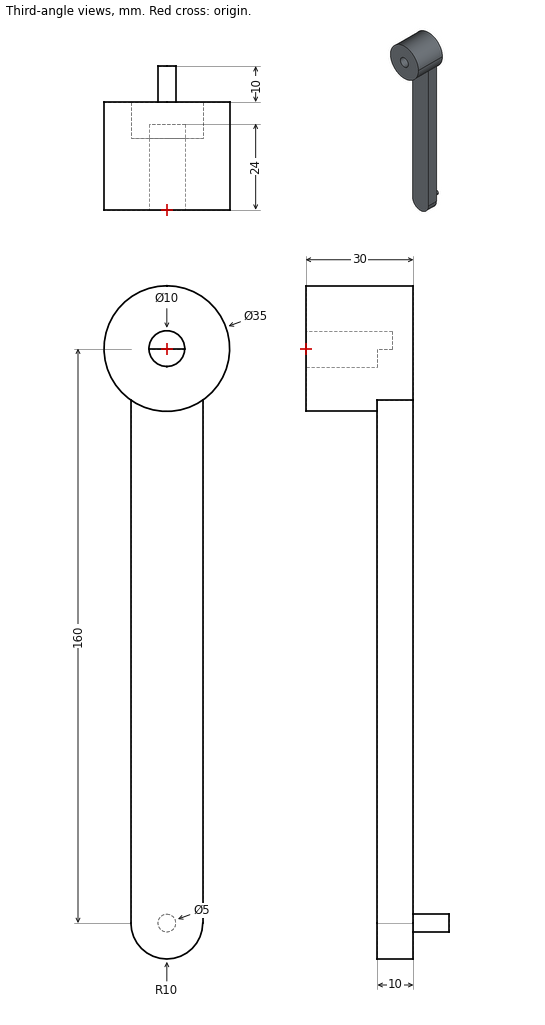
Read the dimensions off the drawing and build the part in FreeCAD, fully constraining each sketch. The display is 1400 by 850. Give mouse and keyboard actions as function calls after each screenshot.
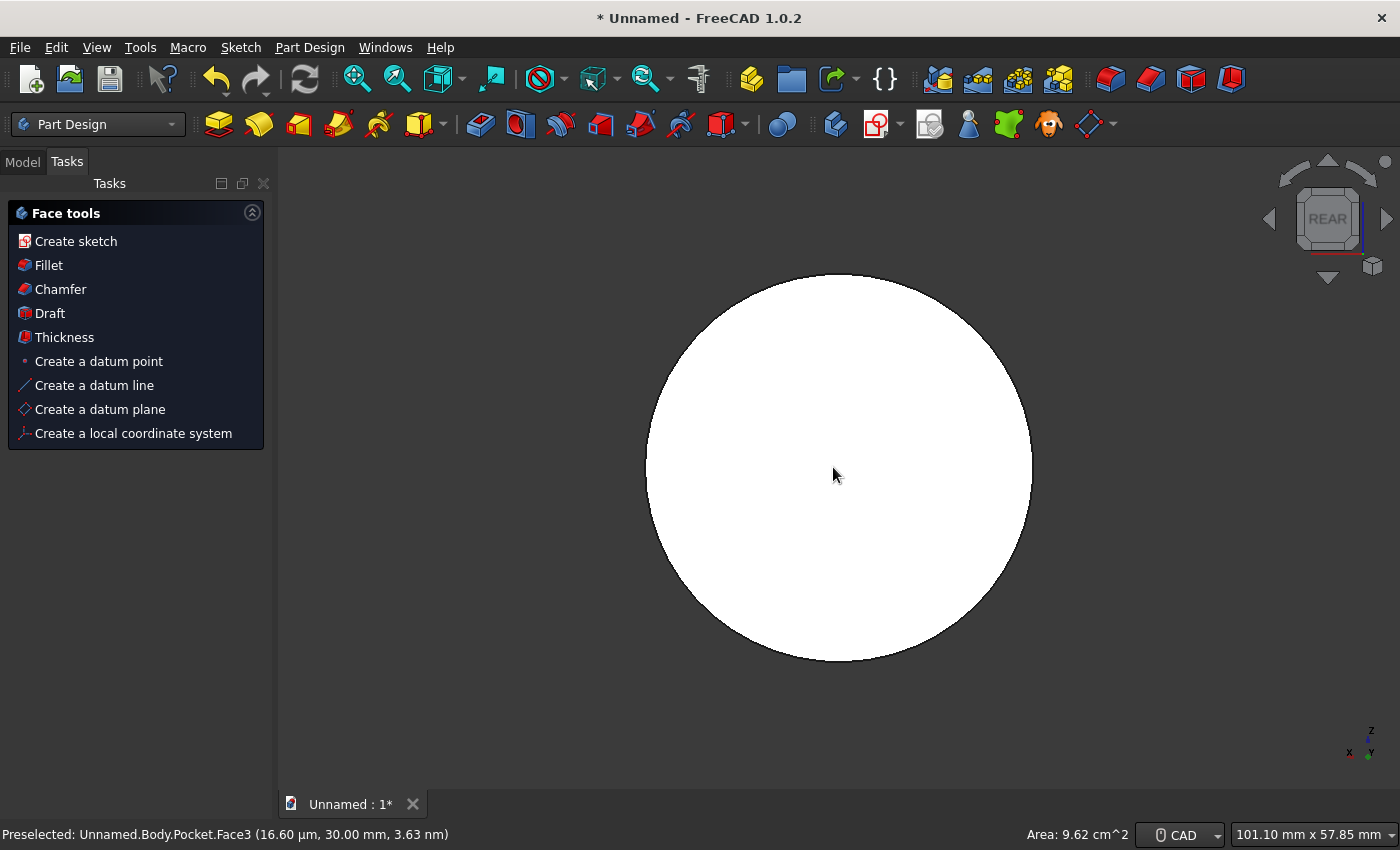
click(876, 124)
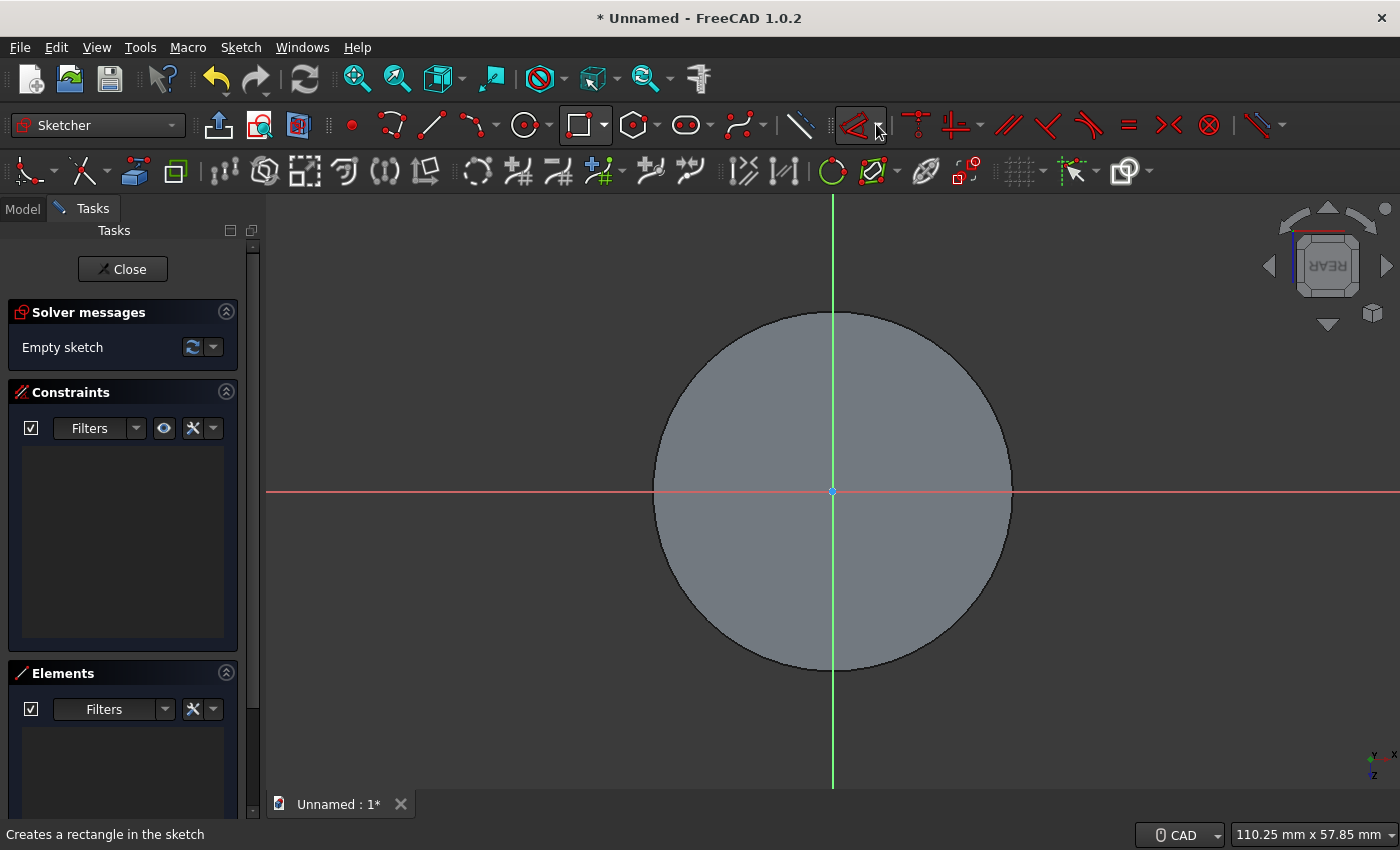
scroll(747, 713, down, 8)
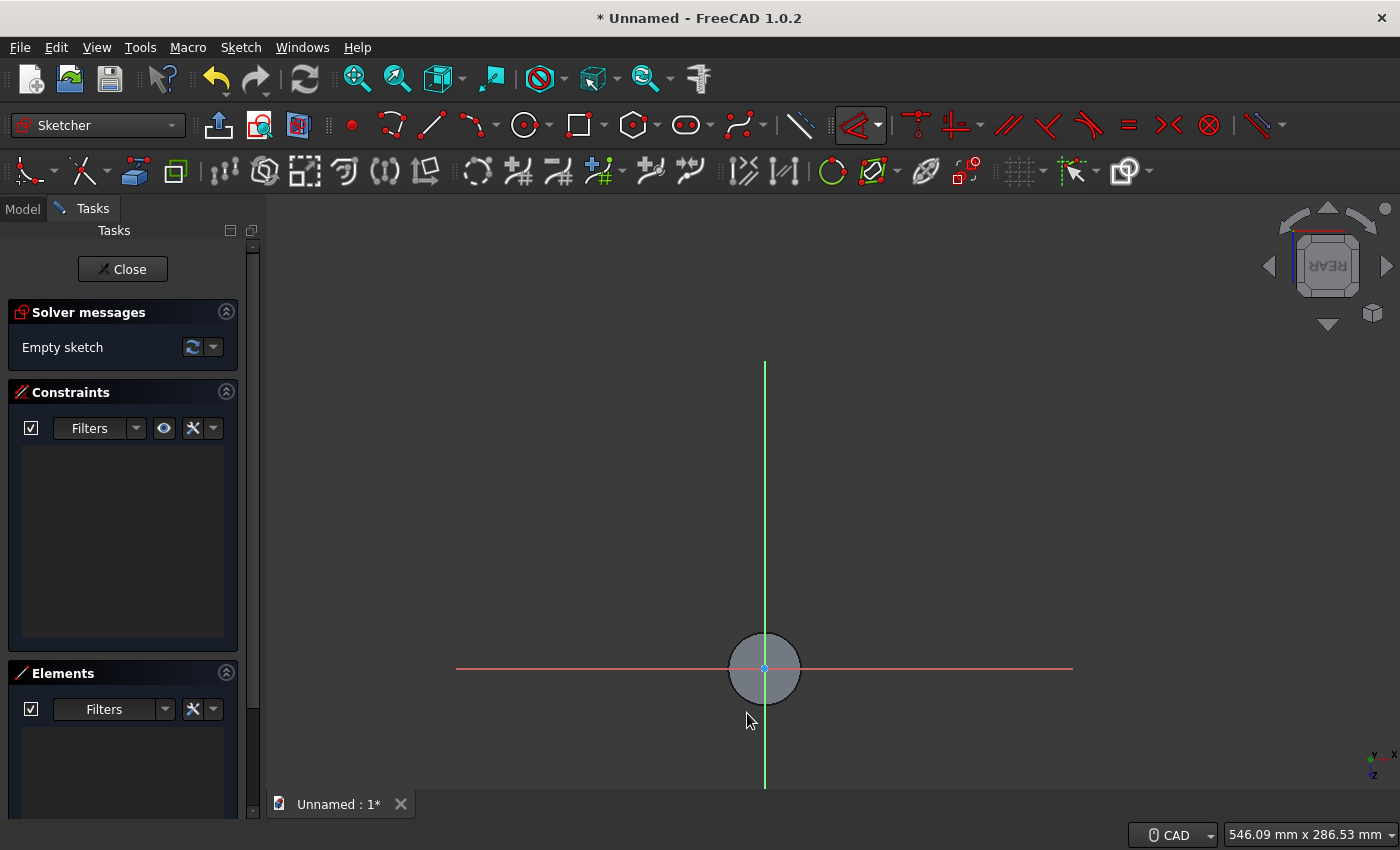
key(g)
key(m)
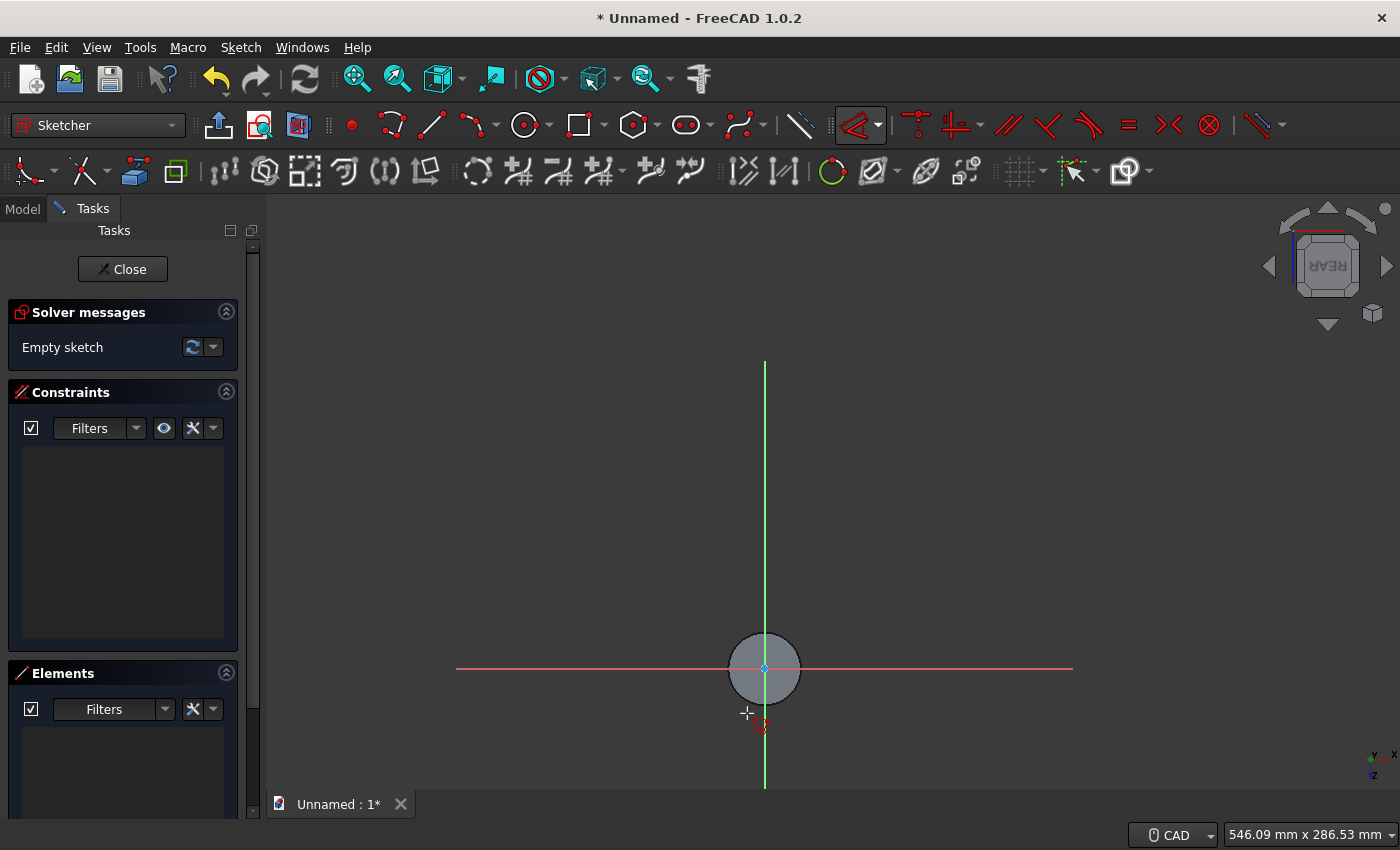
click(744, 337)
click(744, 669)
click(785, 660)
click(785, 337)
right_click(785, 337)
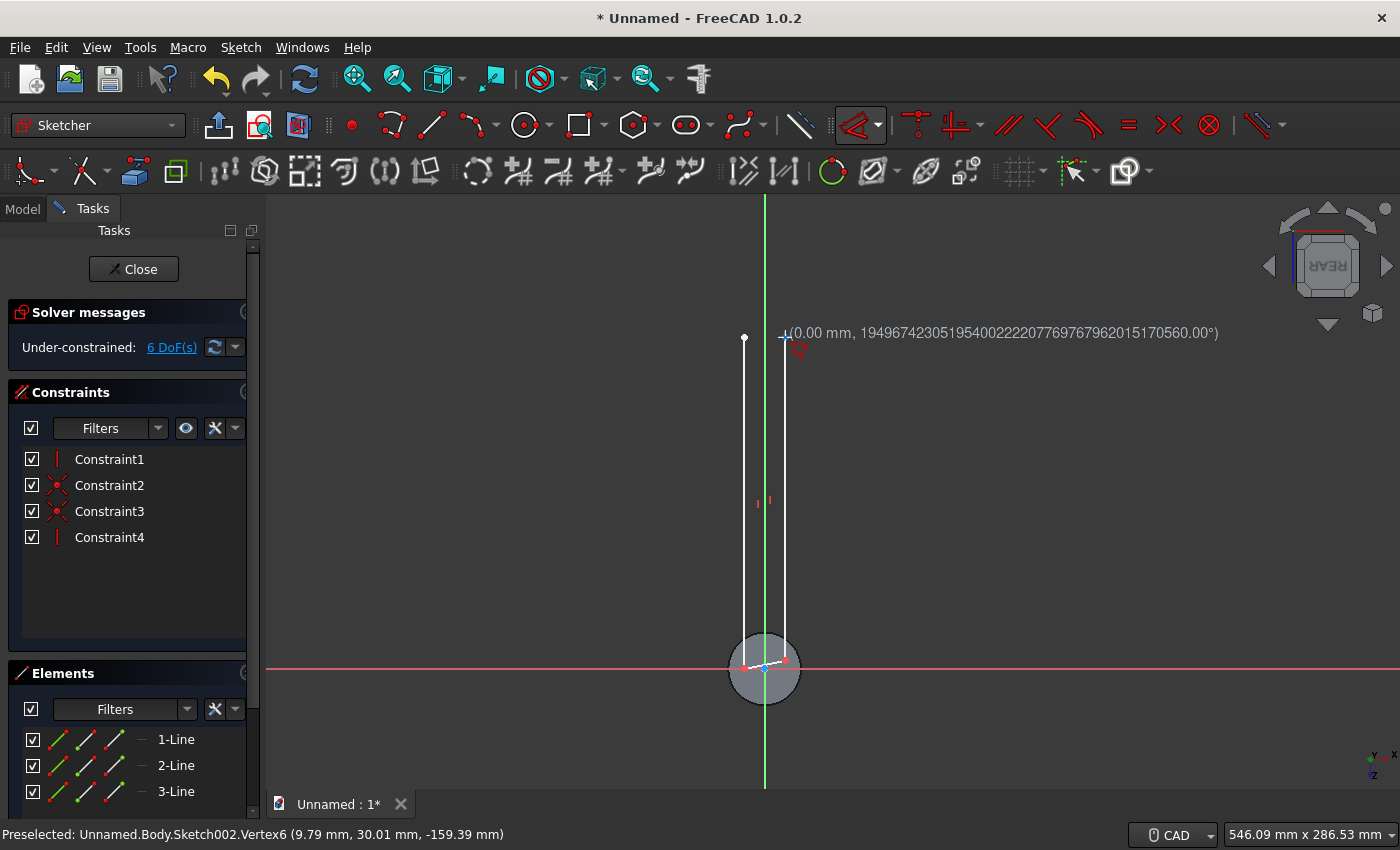
key(g)
key(3)
key(a)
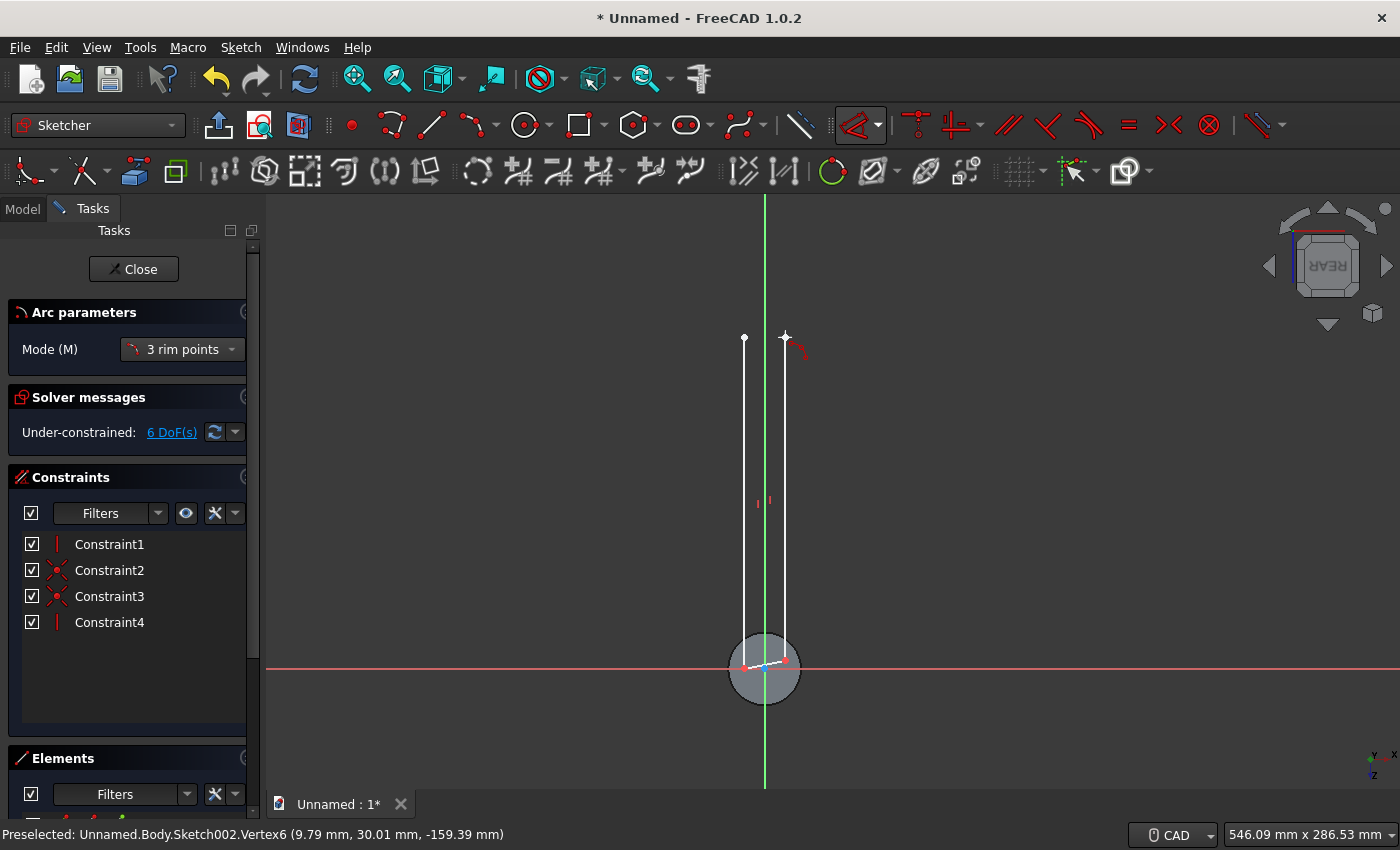
click(785, 338)
click(744, 338)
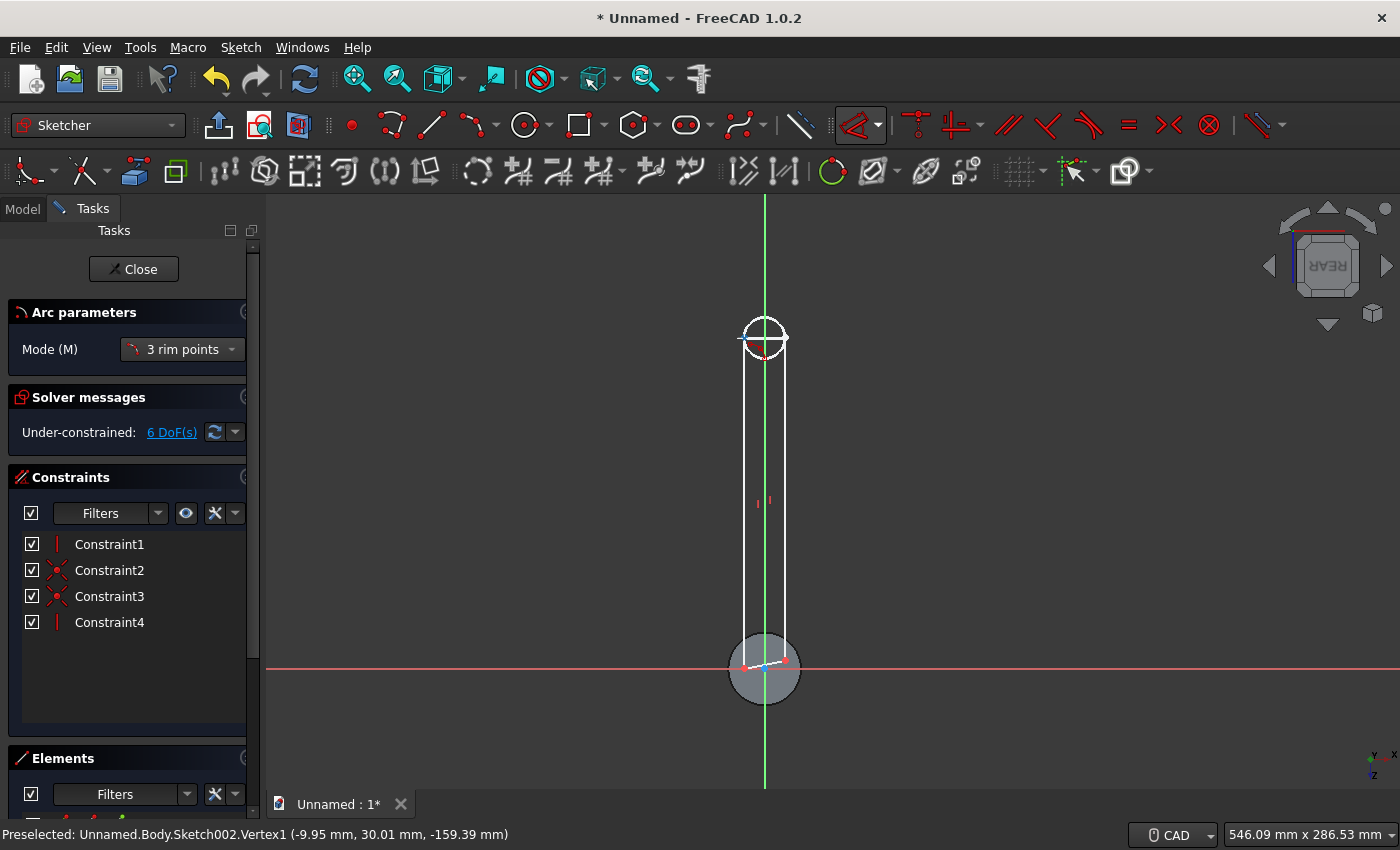
scroll(777, 320, up, 2)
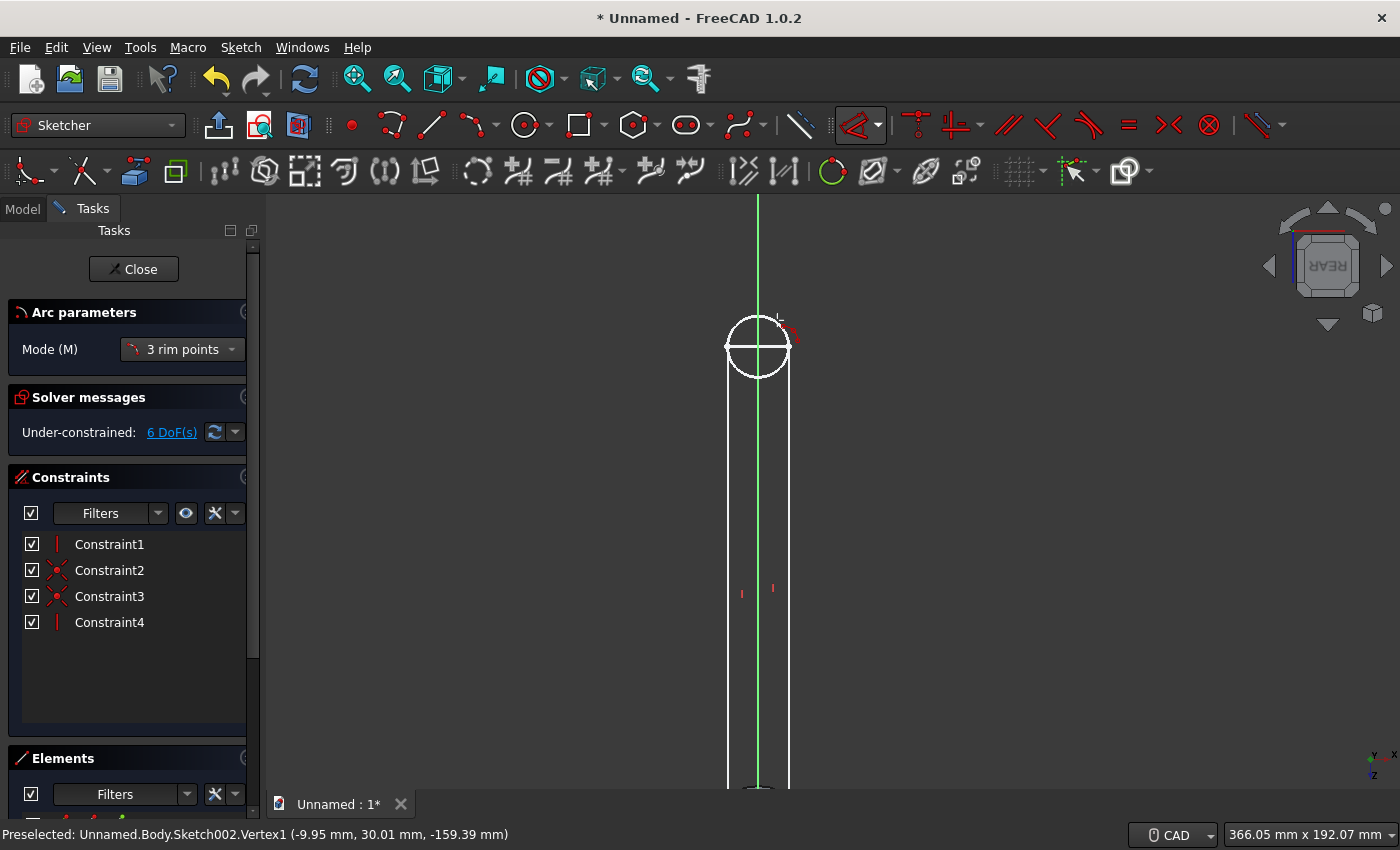
click(777, 320)
key(Escape)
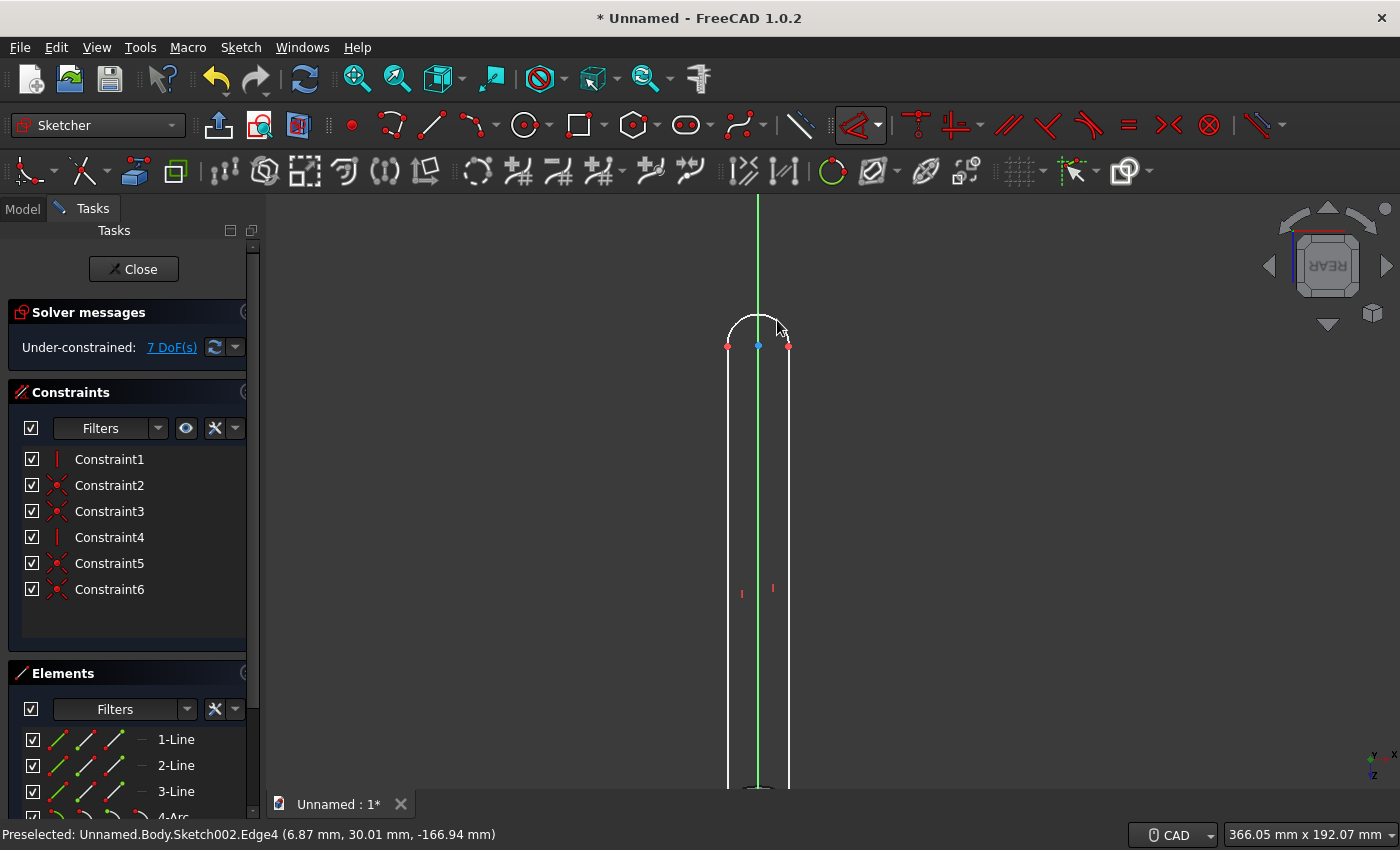
click(728, 495)